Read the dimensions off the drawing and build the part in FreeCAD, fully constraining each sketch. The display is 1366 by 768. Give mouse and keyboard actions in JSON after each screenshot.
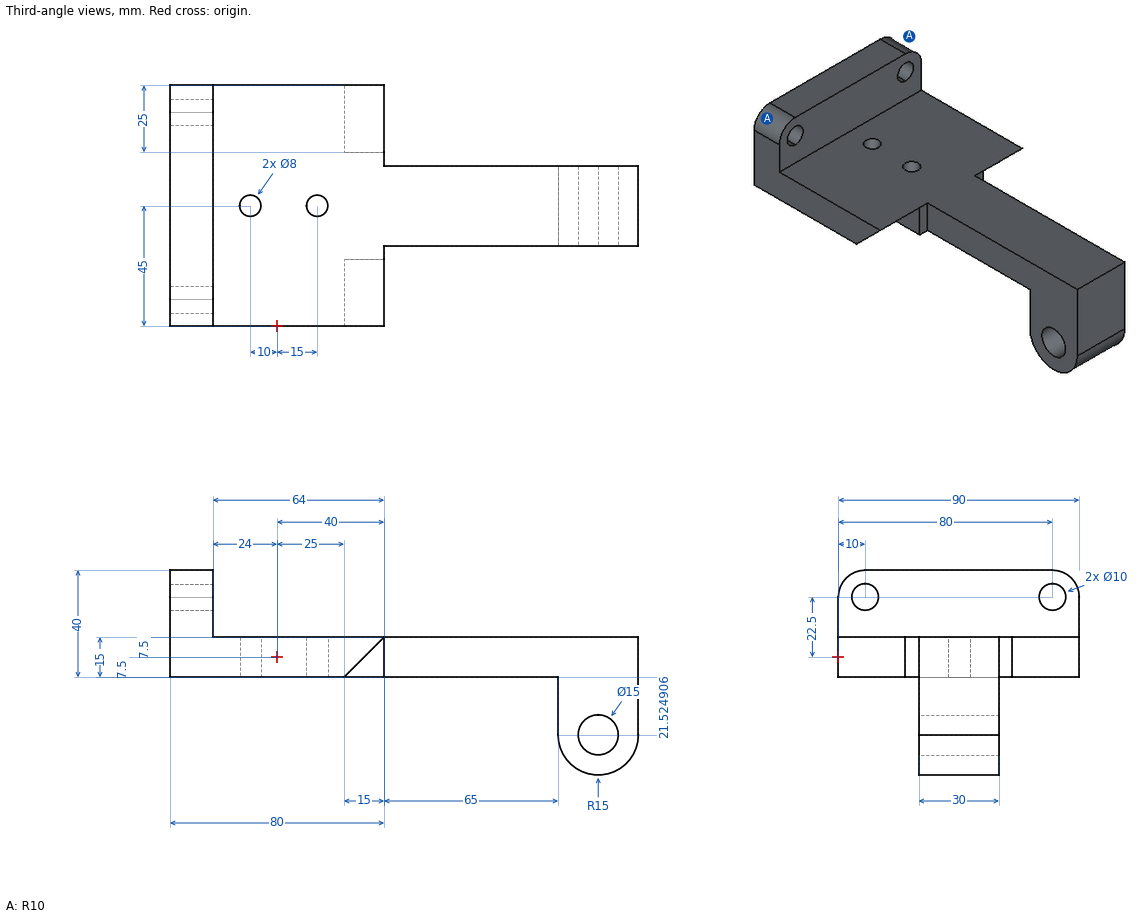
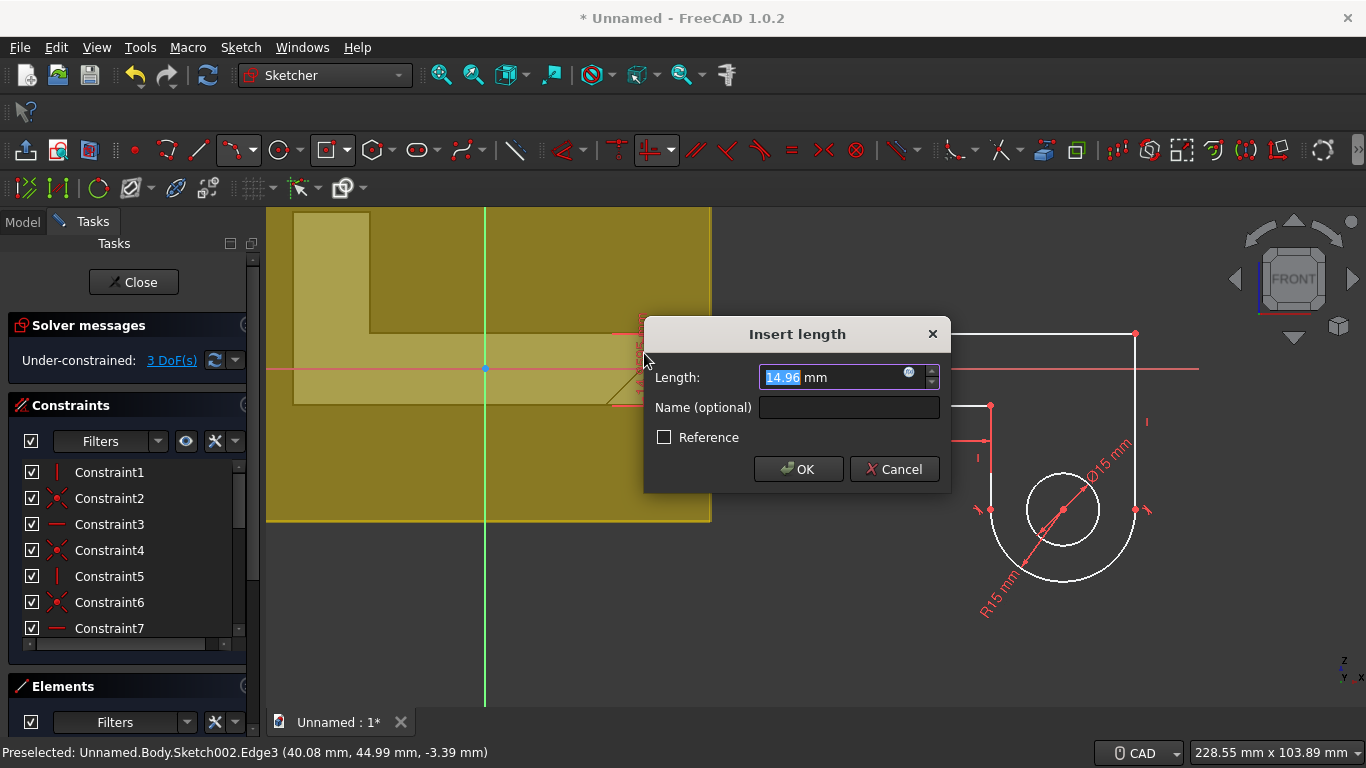
{"action": "type", "text": "15"}
{"action": "key", "text": "Return"}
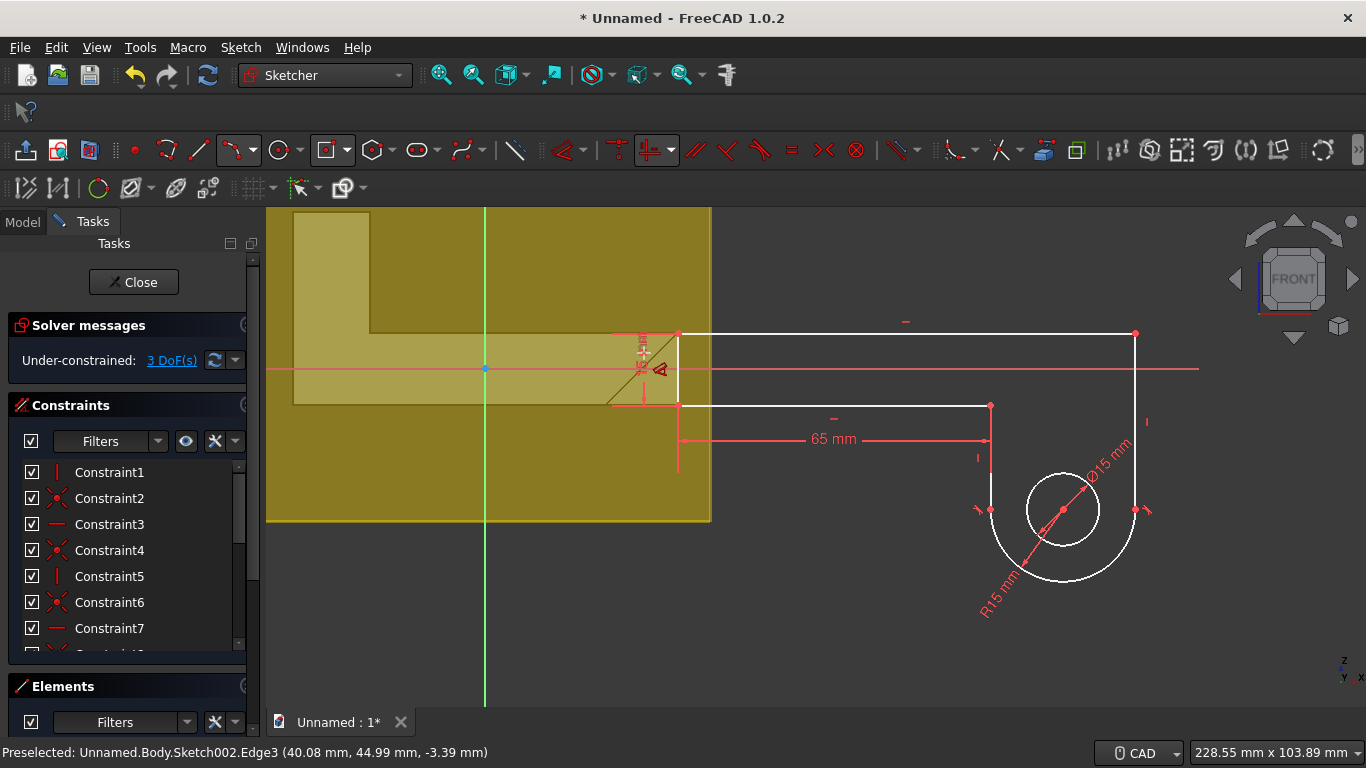
{"action": "left_click", "coordinate": [678, 406]}
{"action": "left_click", "coordinate": [537, 335]}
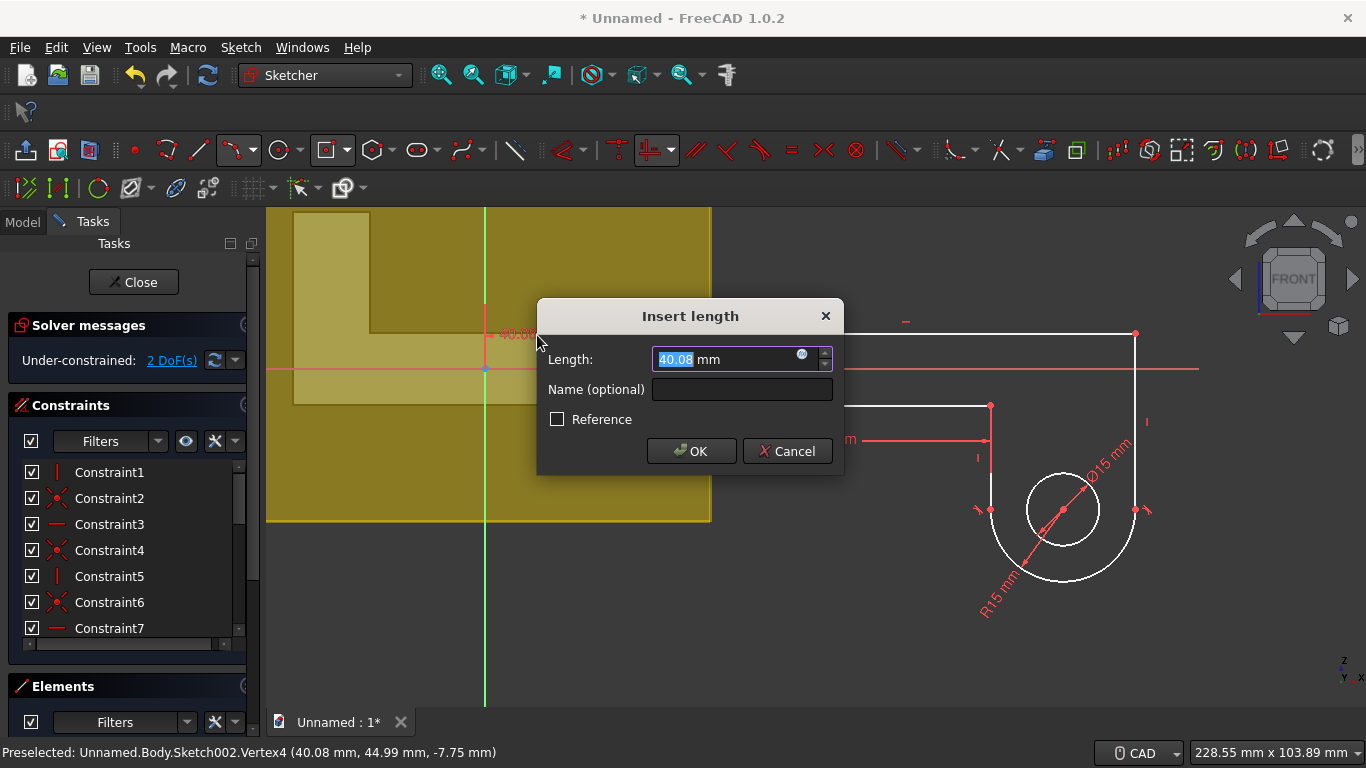
{"action": "type", "text": "40"}
{"action": "key", "text": "Return"}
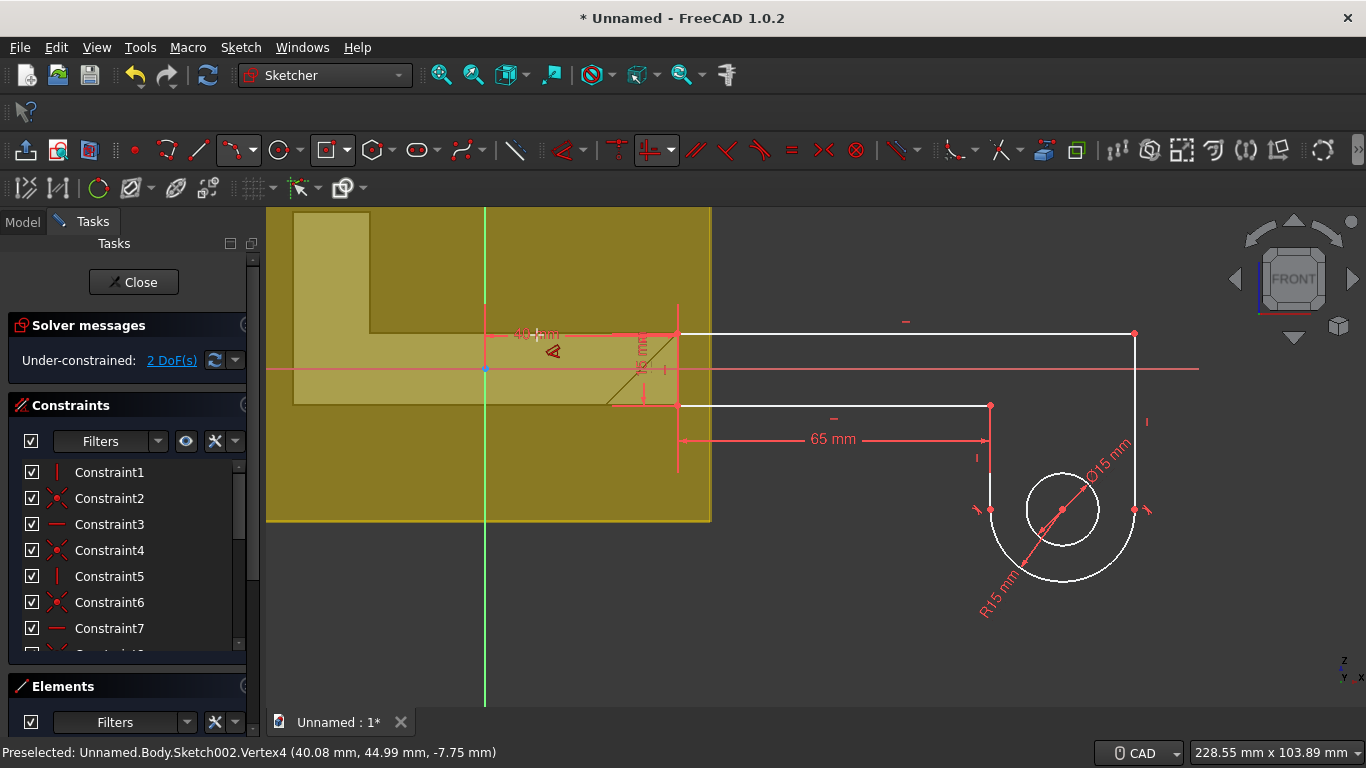
{"action": "left_click", "coordinate": [990, 406]}
{"action": "left_click", "coordinate": [451, 387]}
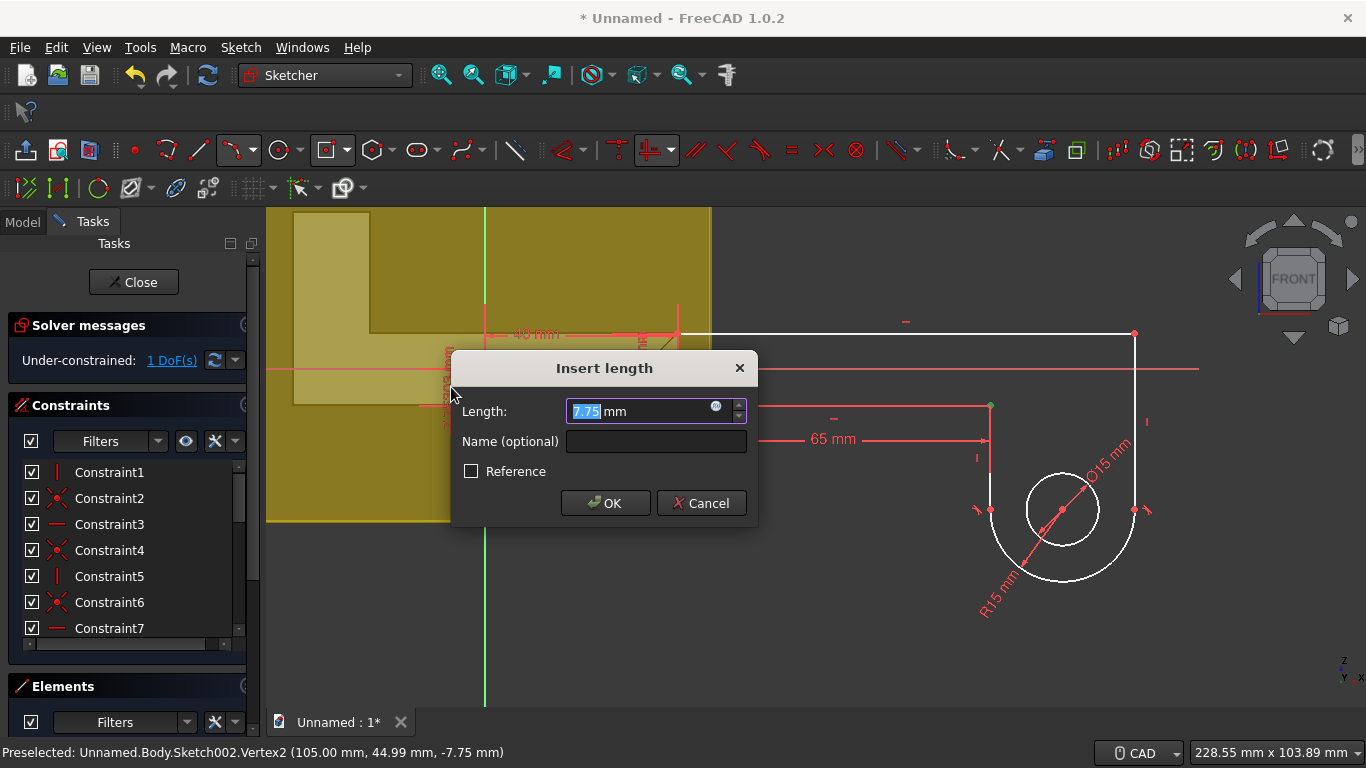
{"action": "type", "text": "7.5"}
{"action": "key", "text": "Return"}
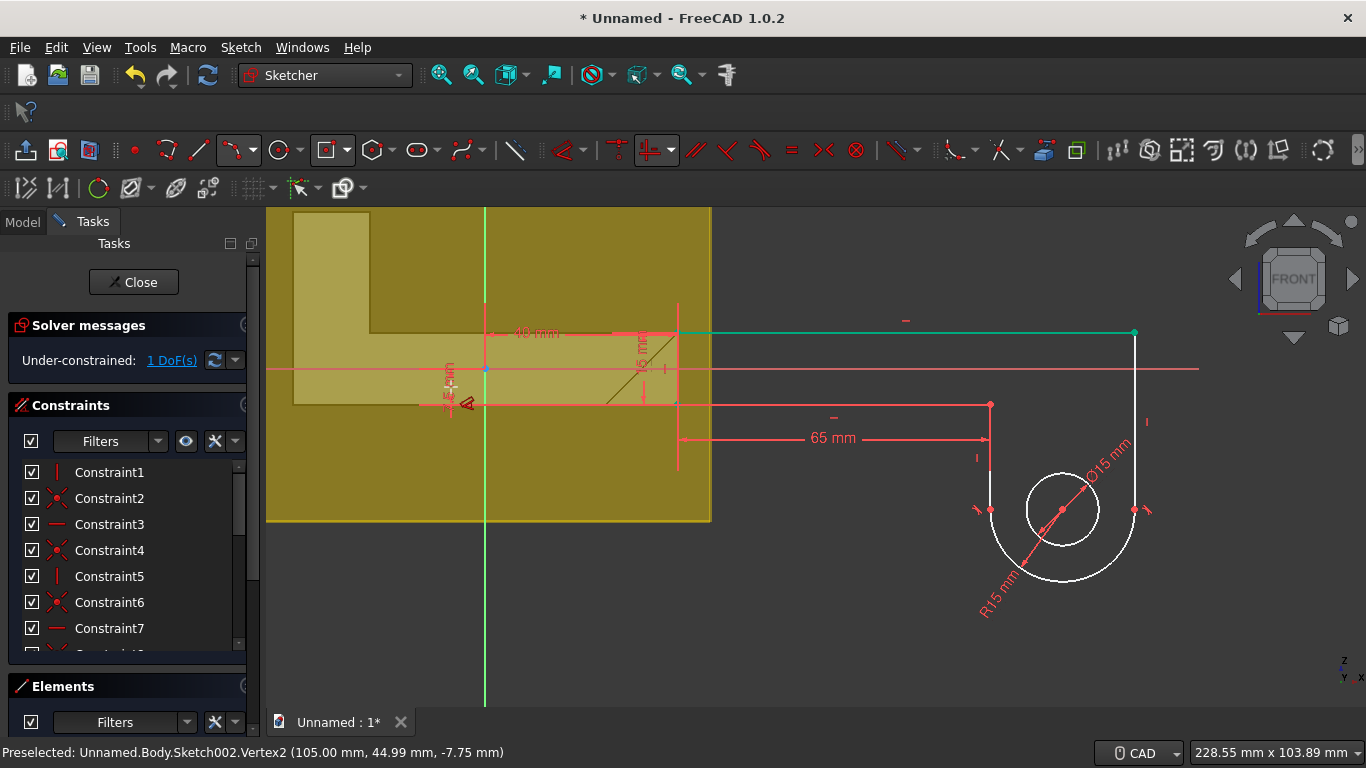
{"action": "left_click", "coordinate": [990, 478]}
{"action": "left_click", "coordinate": [1024, 457]}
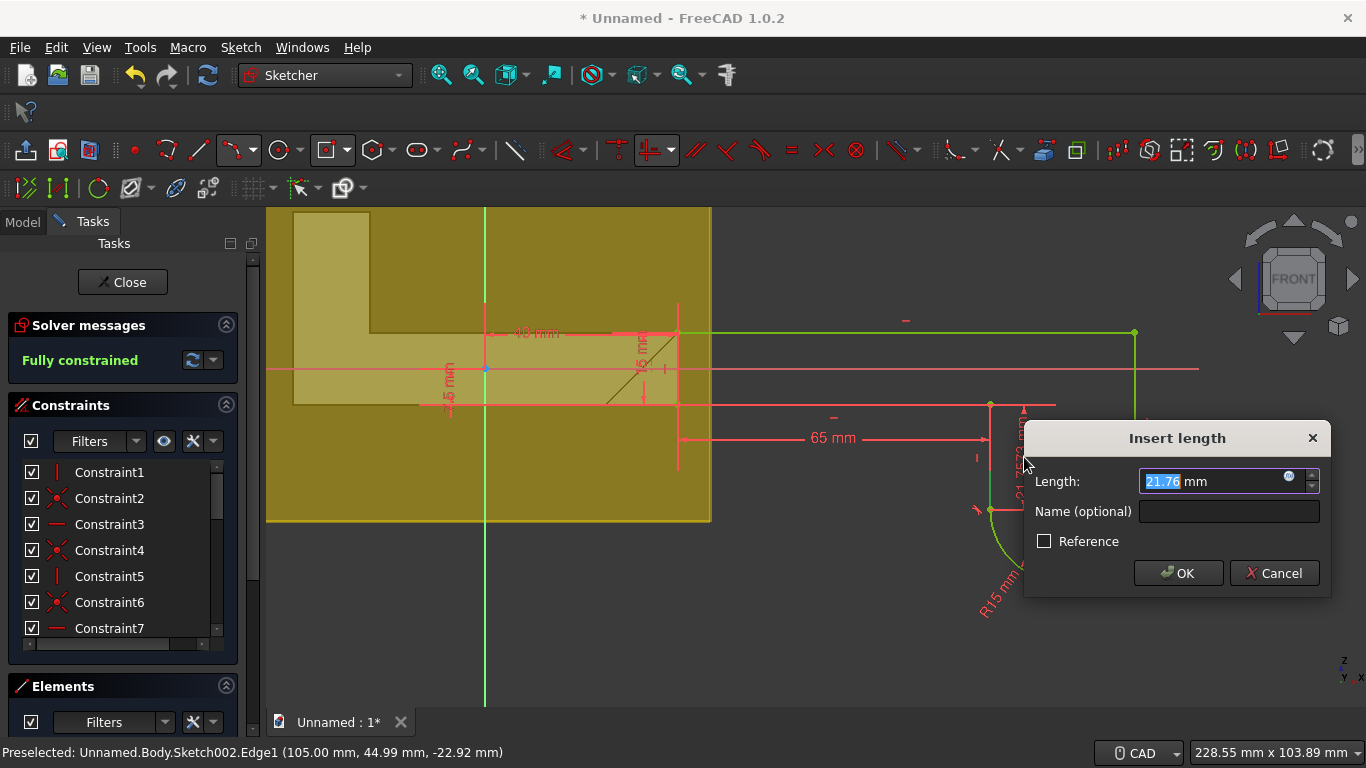
{"action": "type", "text": "21.524906"}
{"action": "key", "text": "Return"}
{"action": "key", "text": "Escape"}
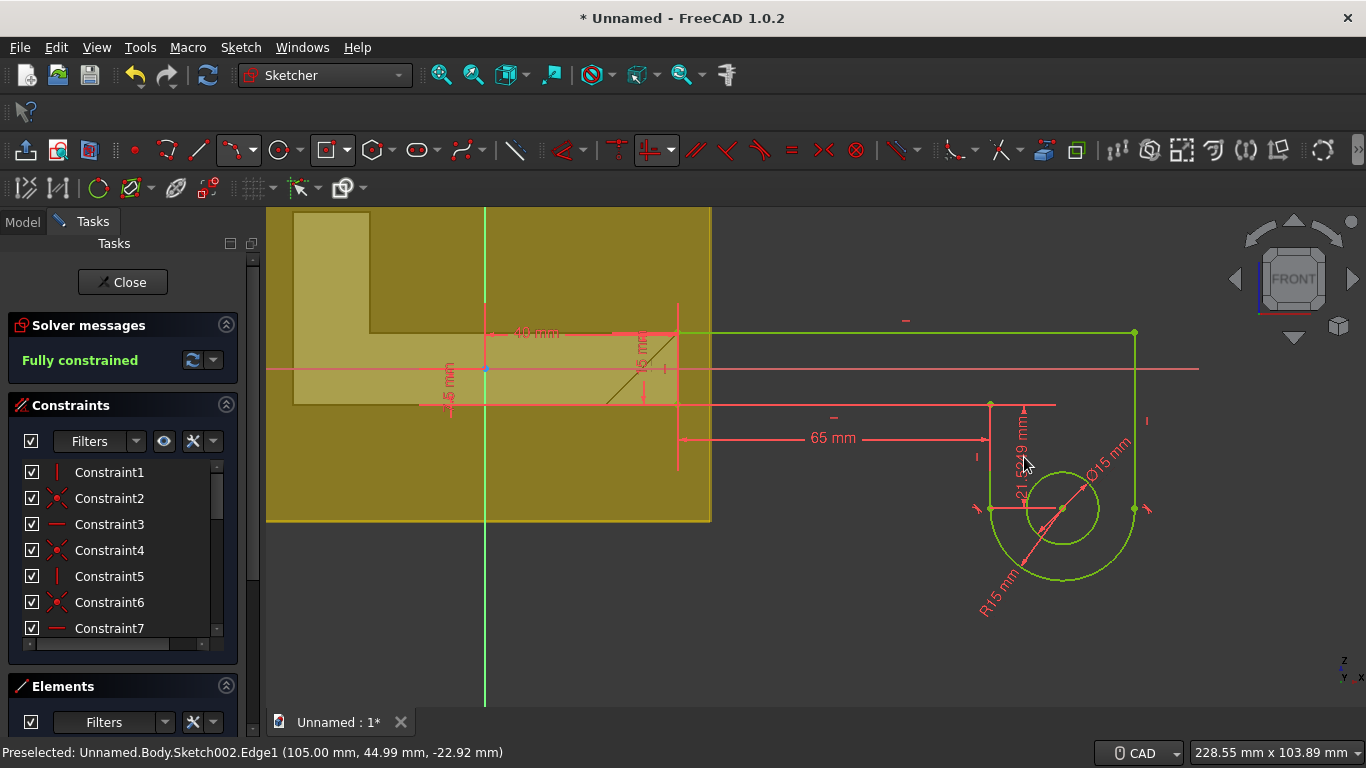
{"action": "left_click", "coordinate": [123, 282]}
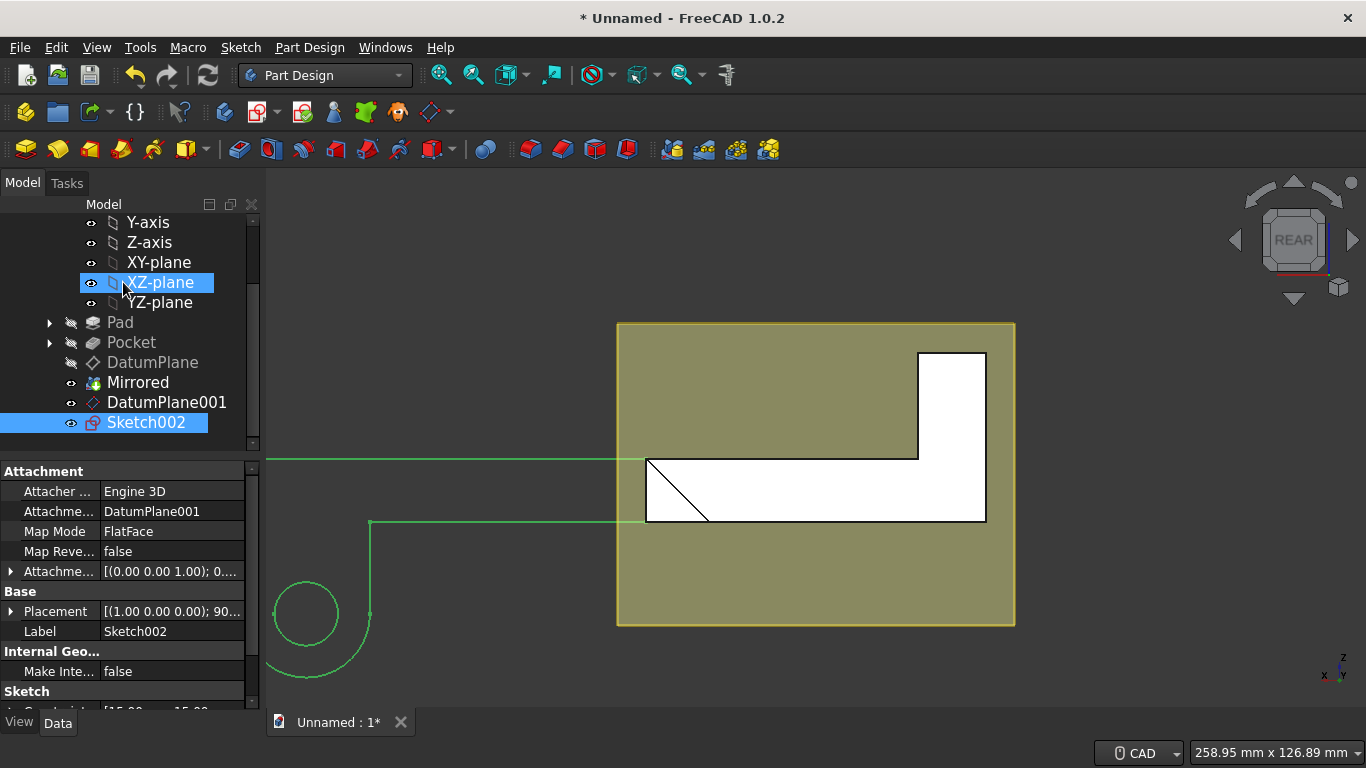
{"action": "left_click", "coordinate": [26, 150]}